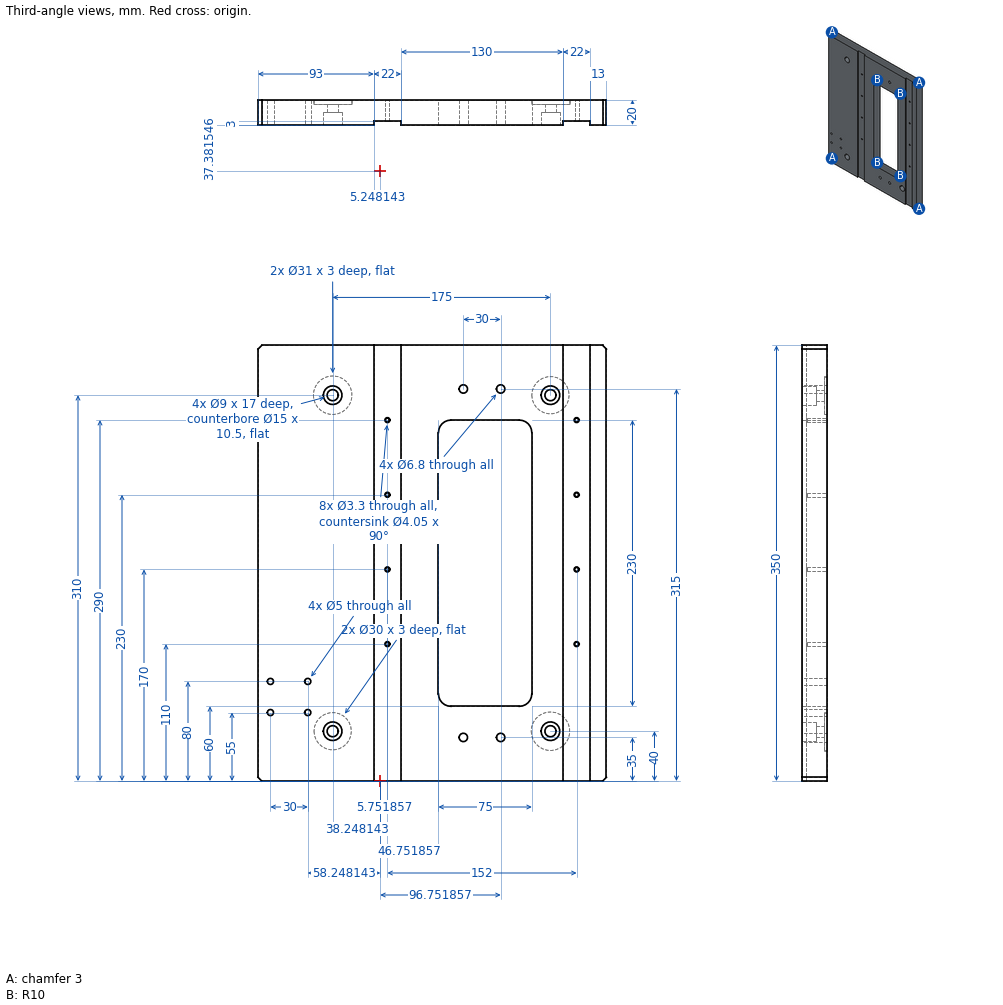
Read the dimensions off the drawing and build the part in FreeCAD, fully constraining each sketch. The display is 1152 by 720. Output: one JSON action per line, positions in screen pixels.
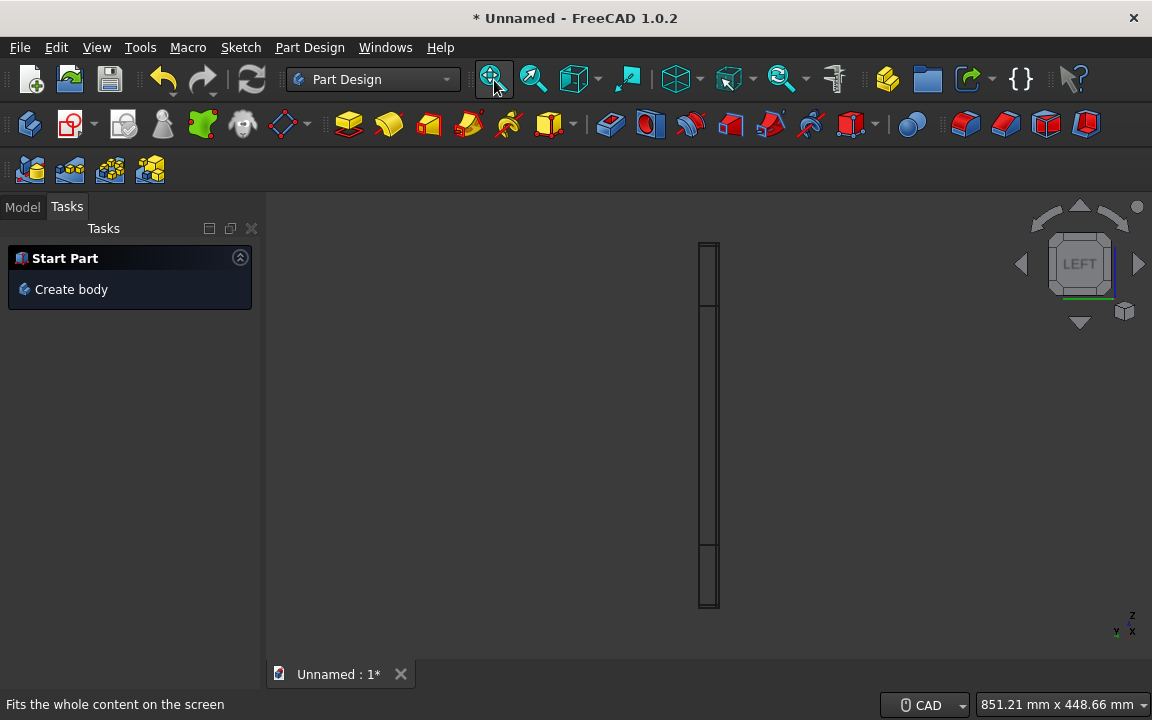
{"action": "key", "text": "0"}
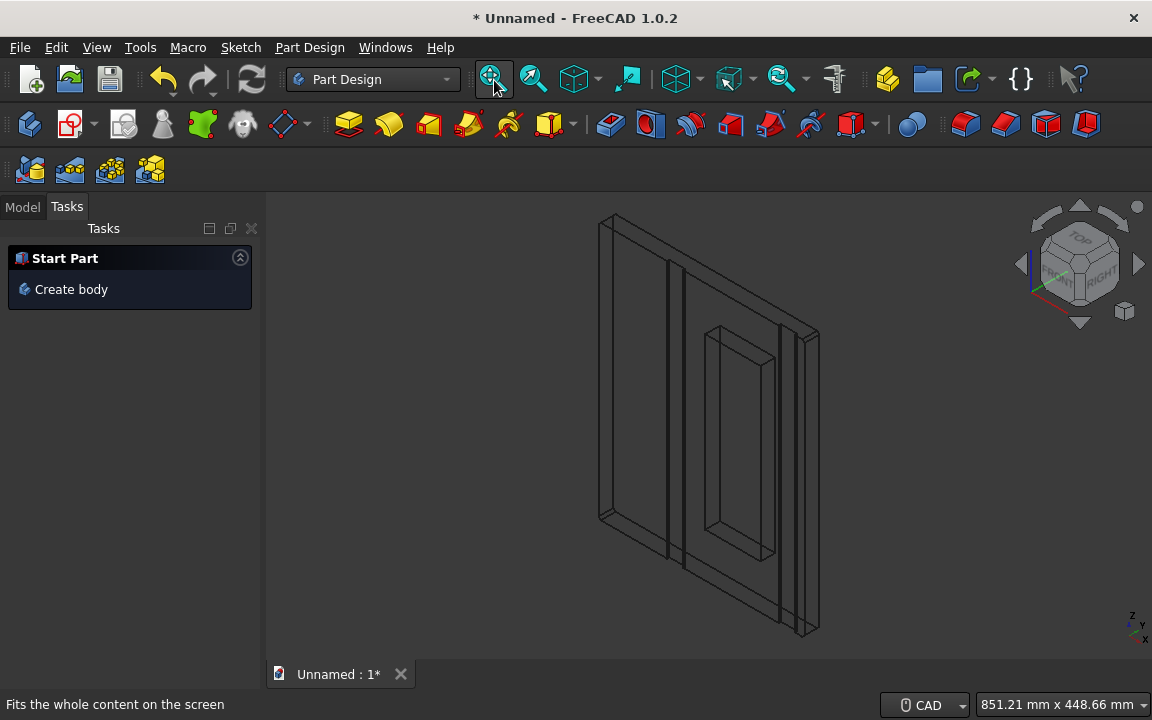
{"action": "left_click", "coordinate": [713, 524]}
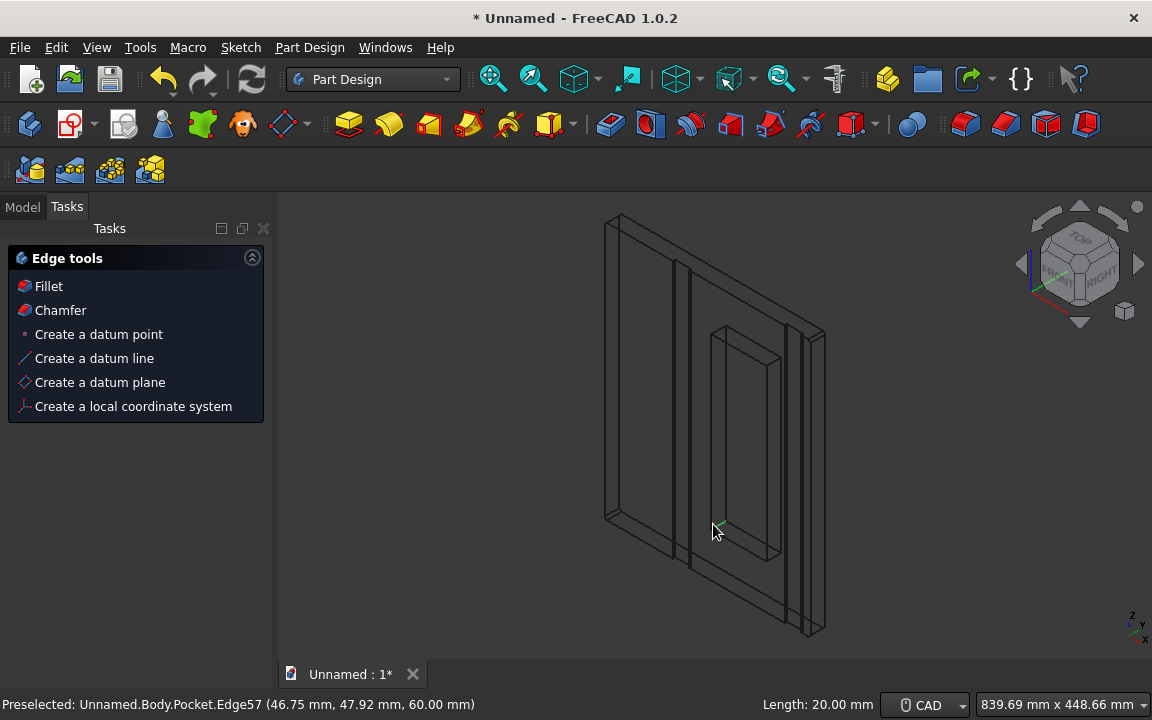
{"action": "left_click", "coordinate": [719, 329], "text": "ctrl"}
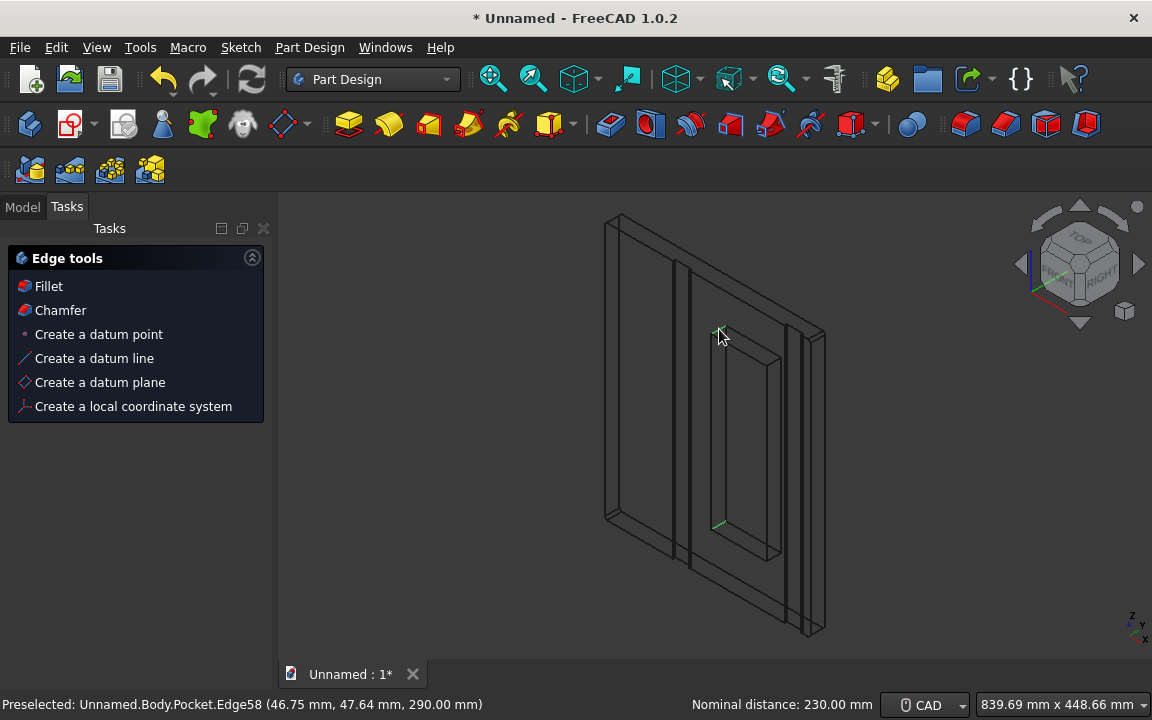
{"action": "left_click", "coordinate": [774, 361], "text": "ctrl"}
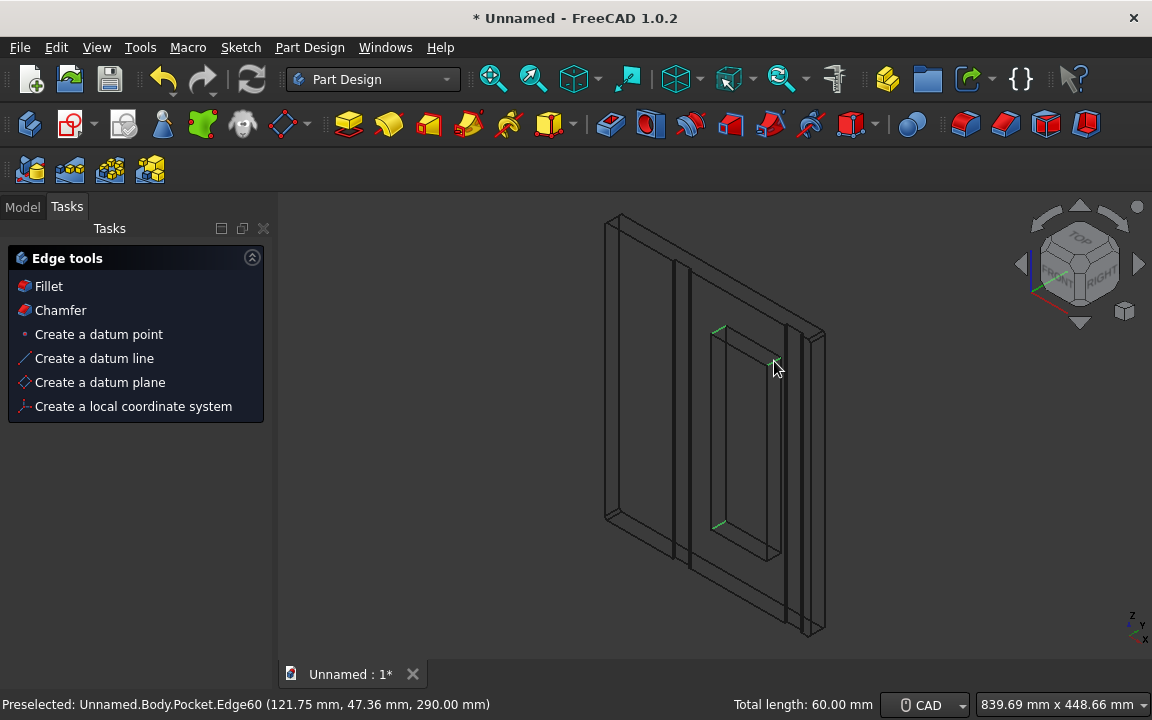
{"action": "left_click", "coordinate": [774, 556], "text": "ctrl"}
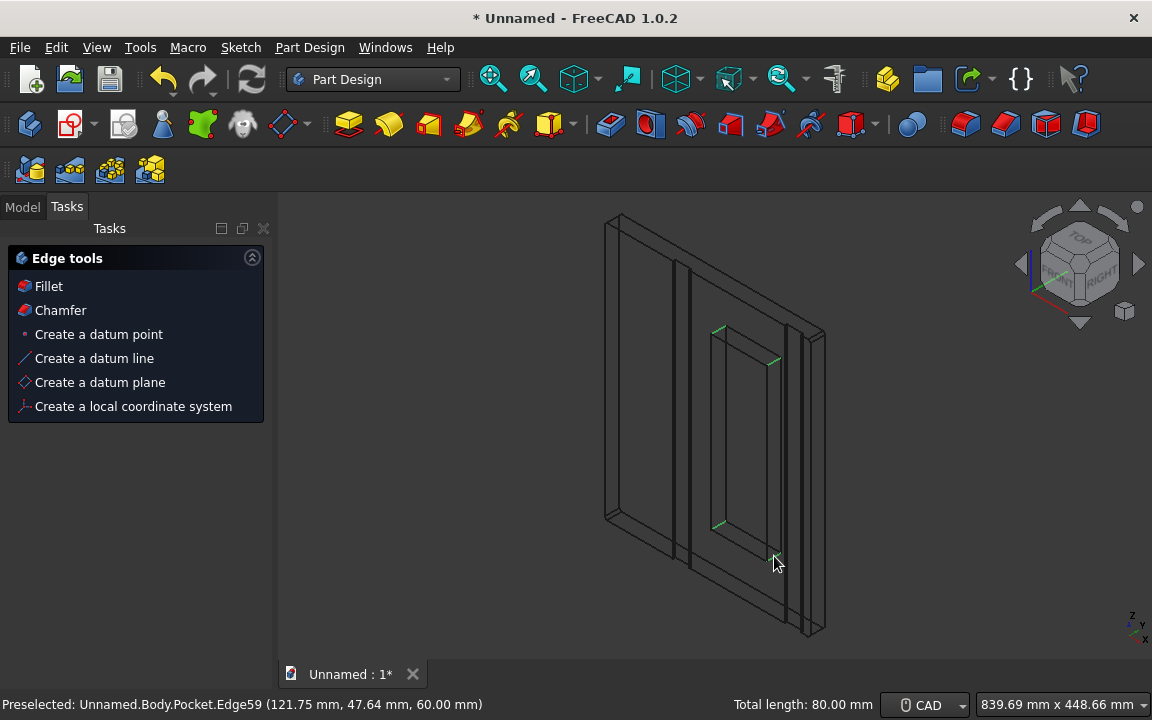
{"action": "key", "text": "v 1"}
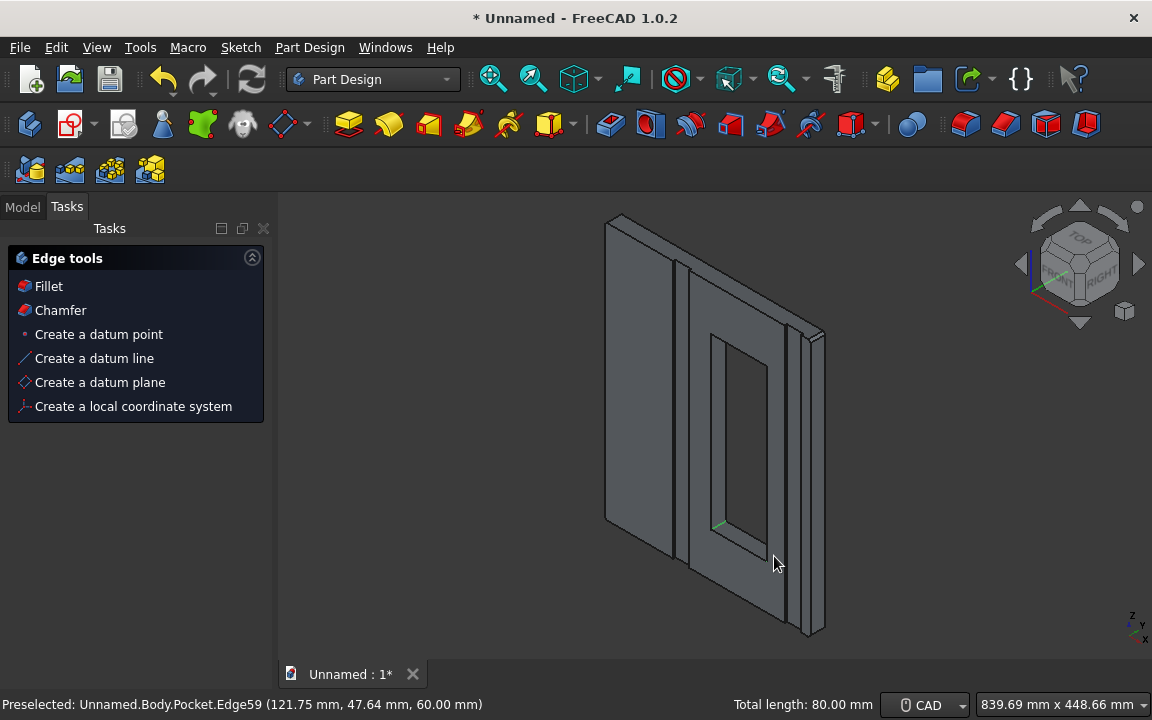
{"action": "left_click", "coordinate": [966, 124]}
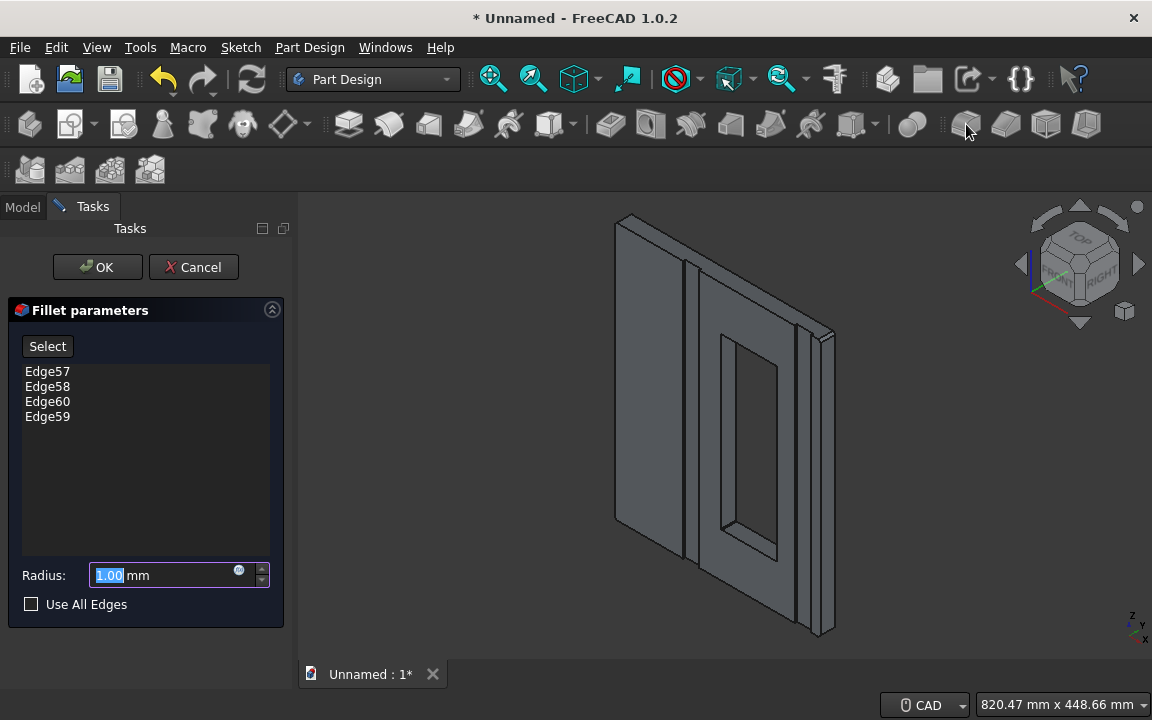
{"action": "type", "text": "10"}
{"action": "key", "text": "Tab"}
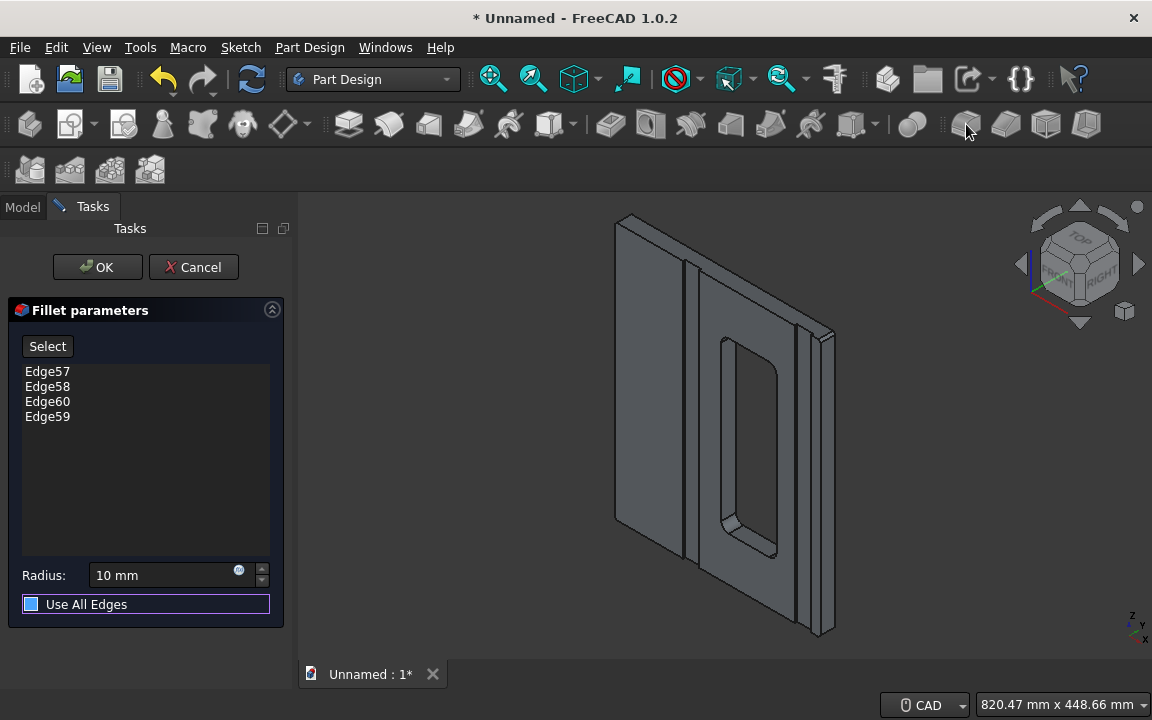
{"action": "left_click", "coordinate": [98, 267]}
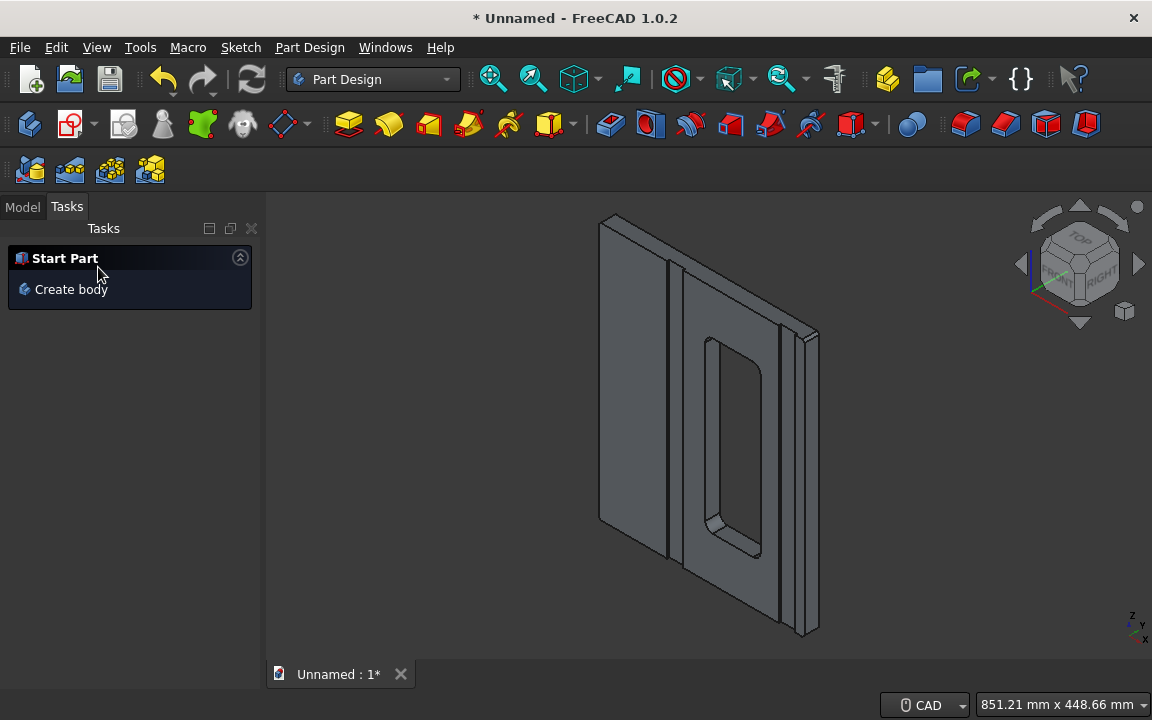
{"action": "left_click", "coordinate": [633, 304]}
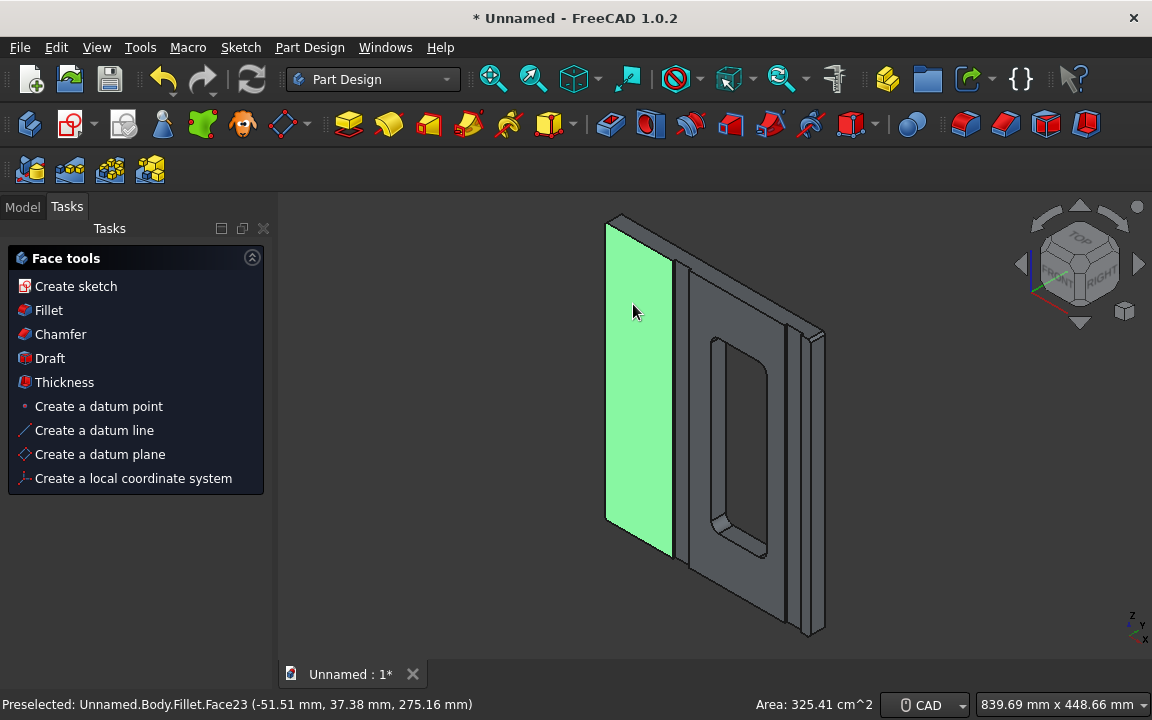
{"action": "left_click", "coordinate": [70, 124]}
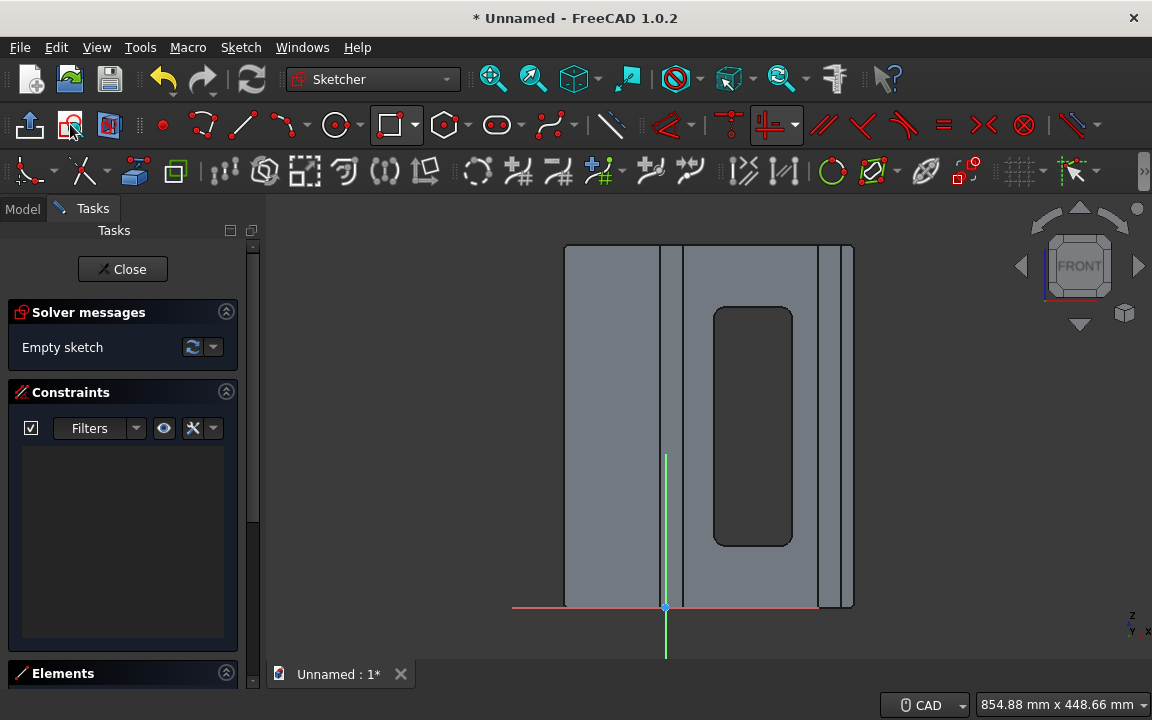
{"action": "scroll", "coordinate": [296, 343], "scroll_direction": "down", "scroll_amount": 1}